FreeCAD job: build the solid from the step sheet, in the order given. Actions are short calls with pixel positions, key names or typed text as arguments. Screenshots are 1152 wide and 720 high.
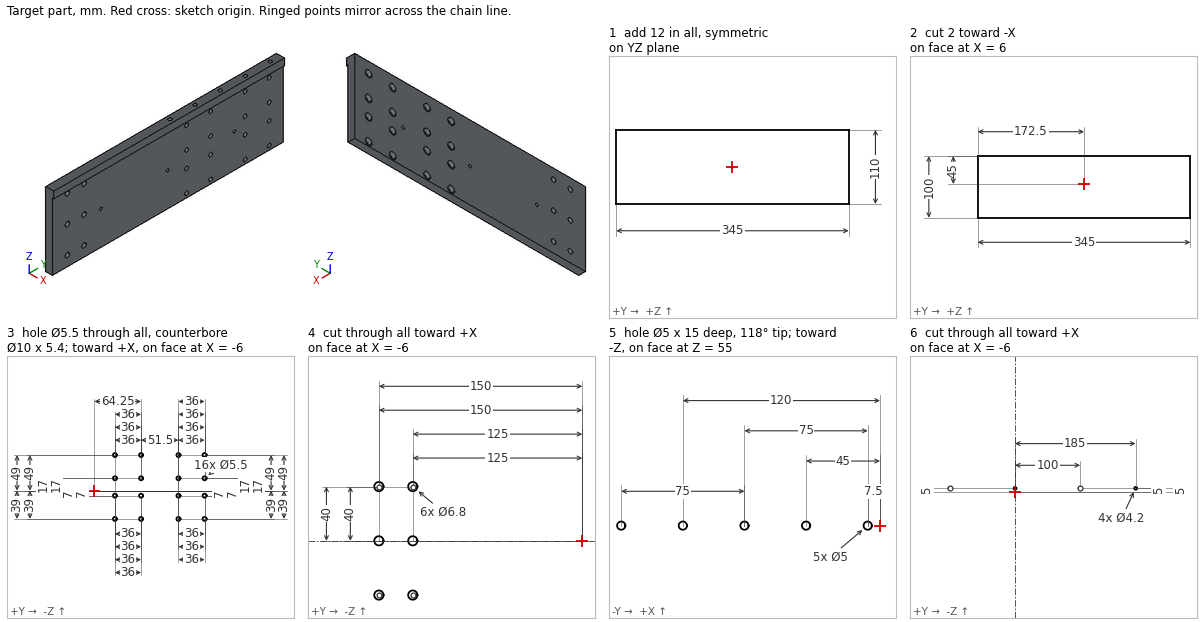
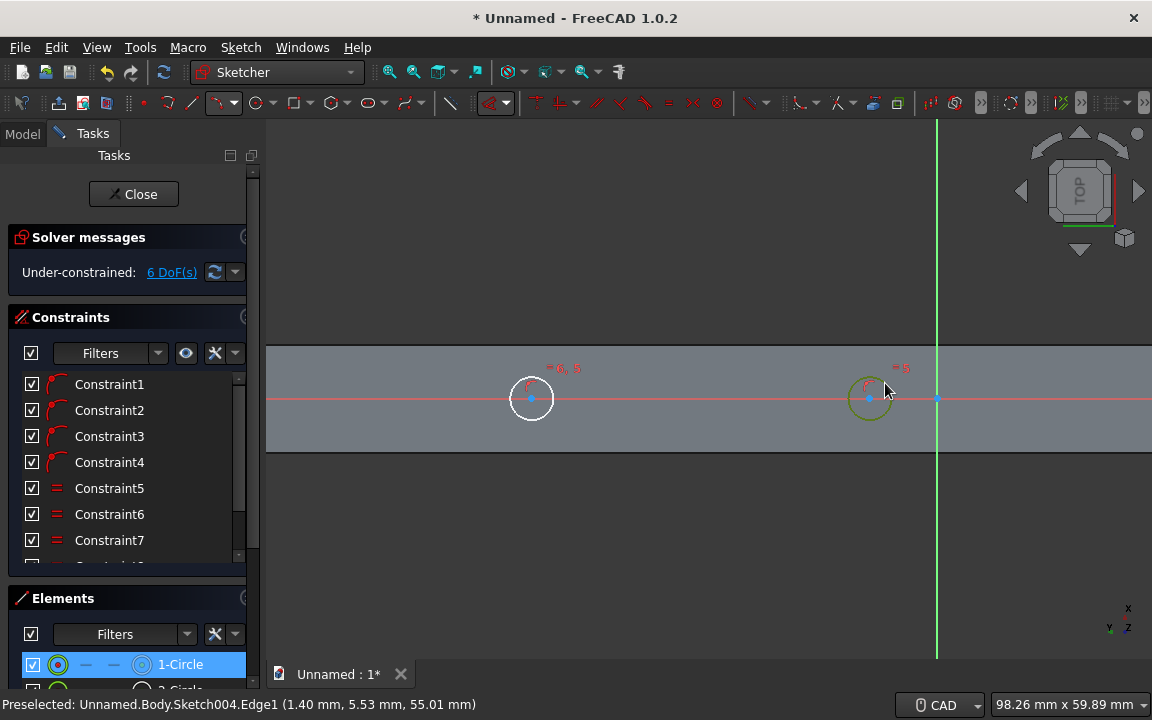
click(508, 104)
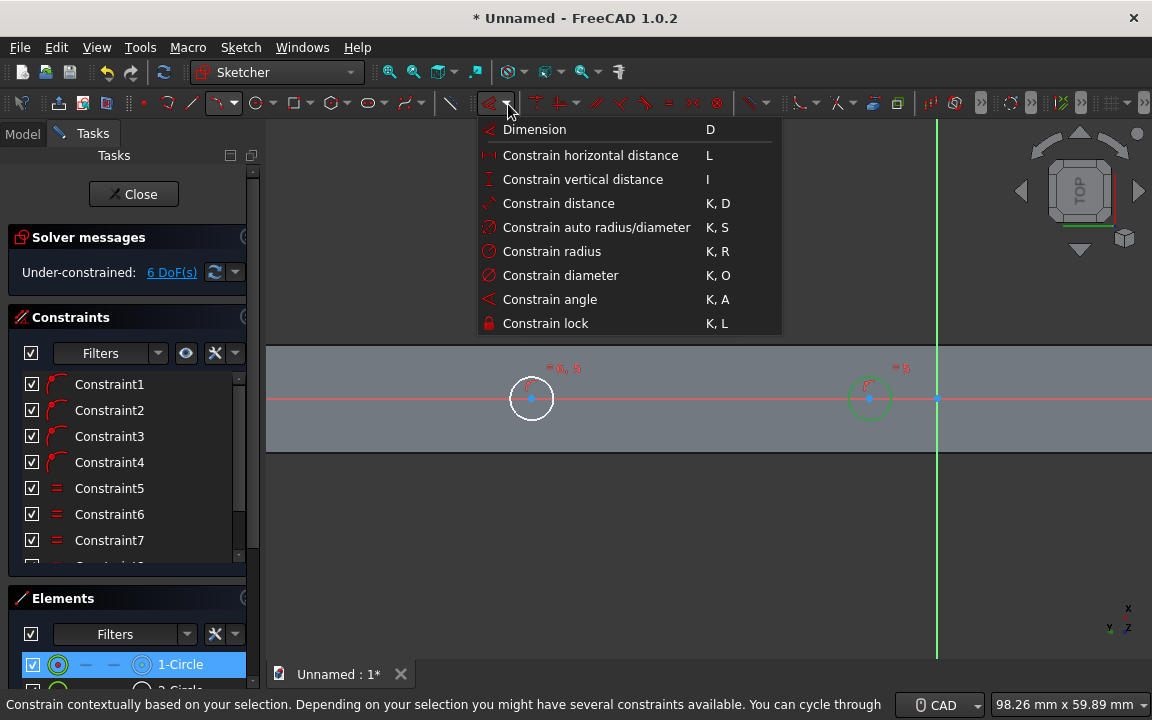
click(630, 275)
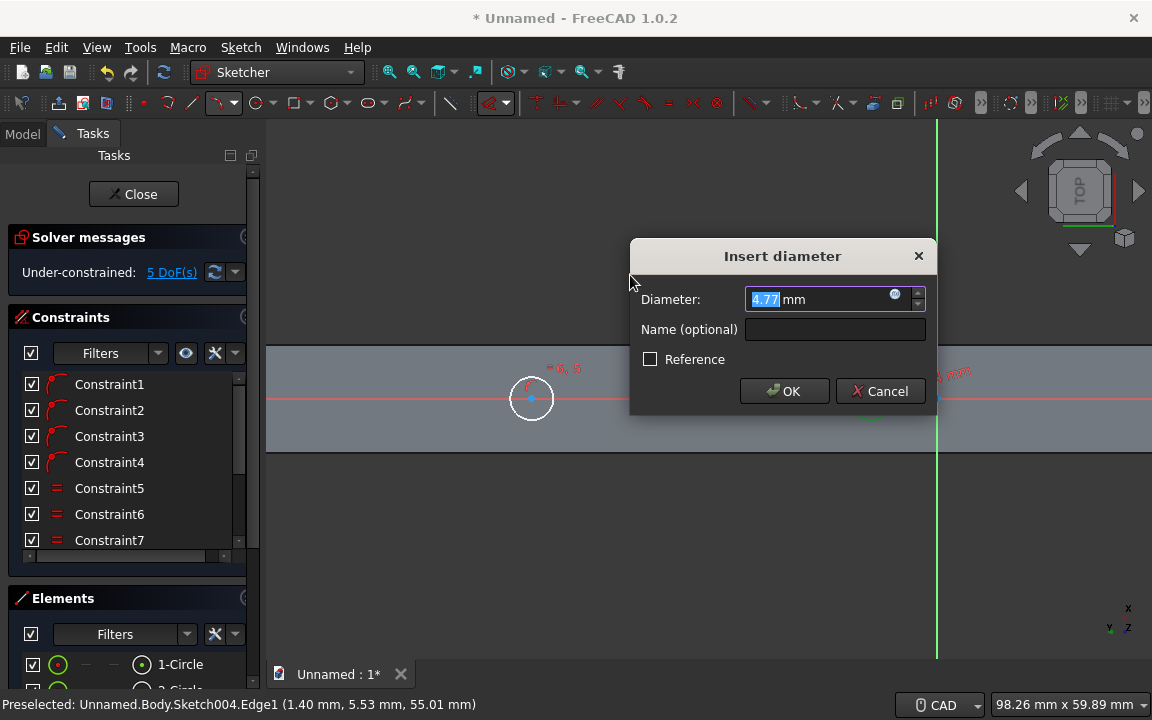
text(5)
key(Return)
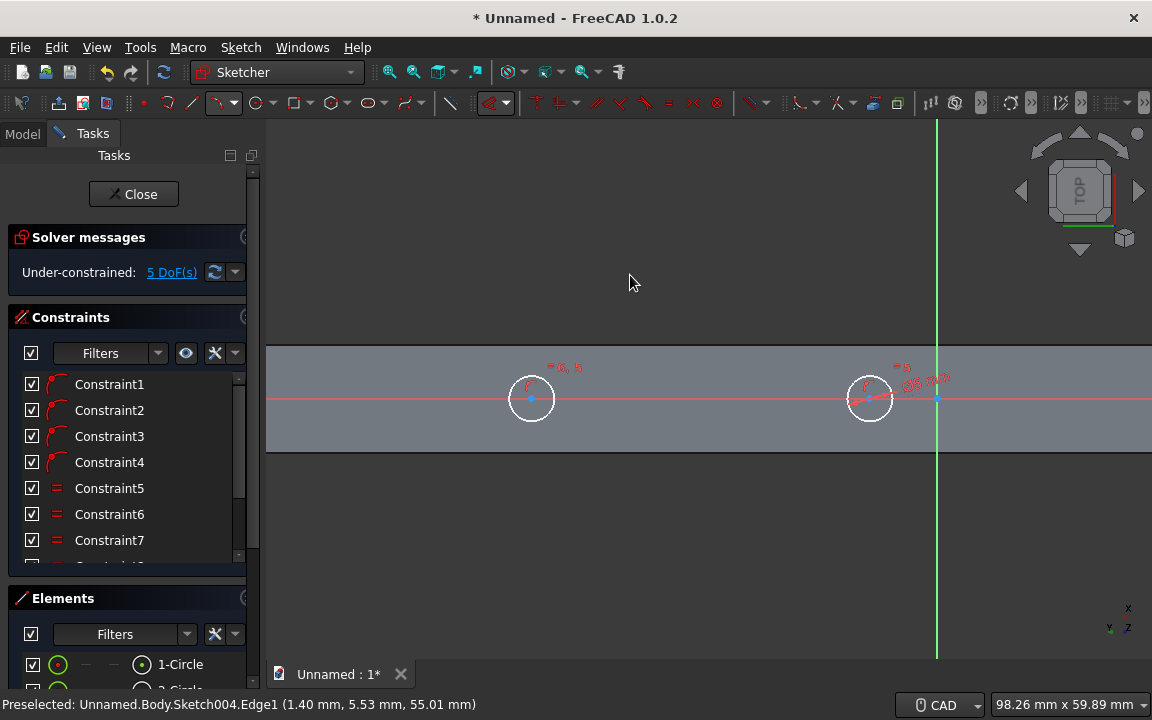
click(532, 399)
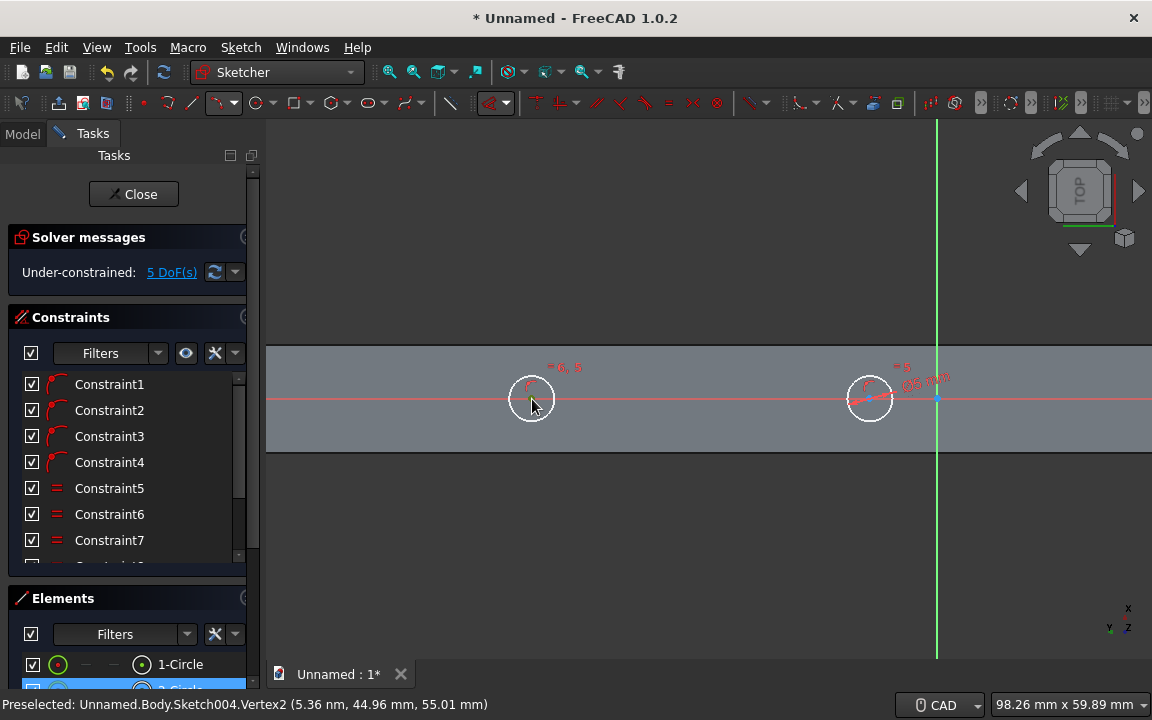
key(l)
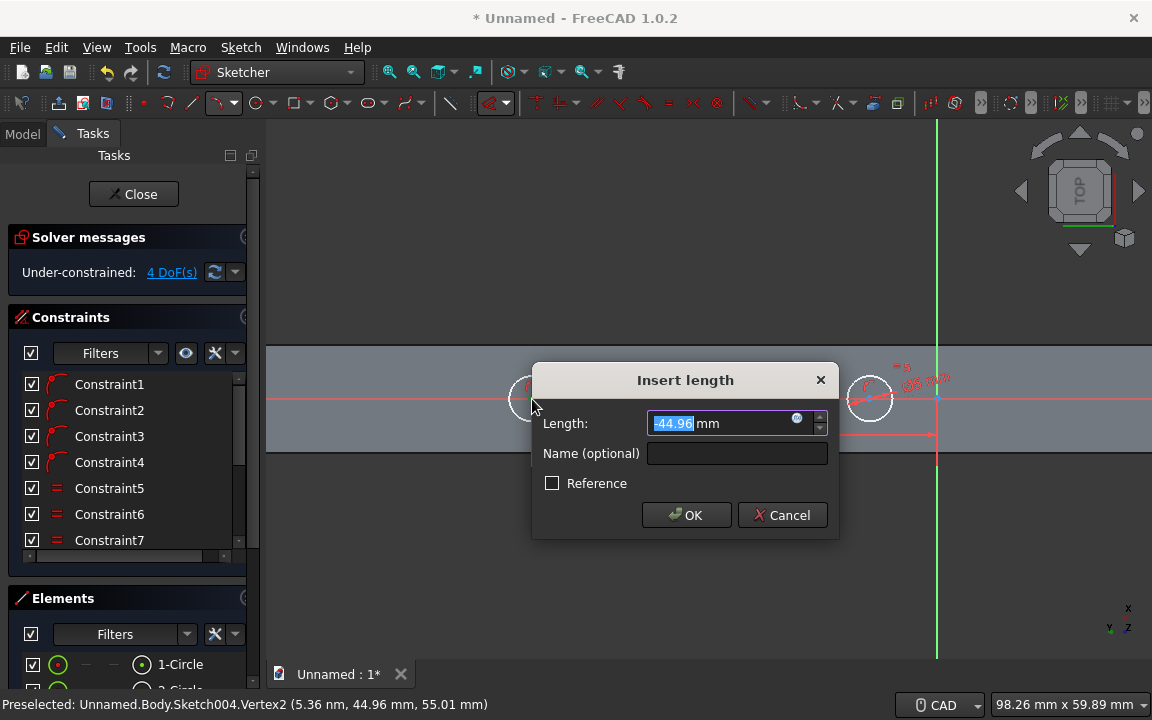
text(-45)
key(Return)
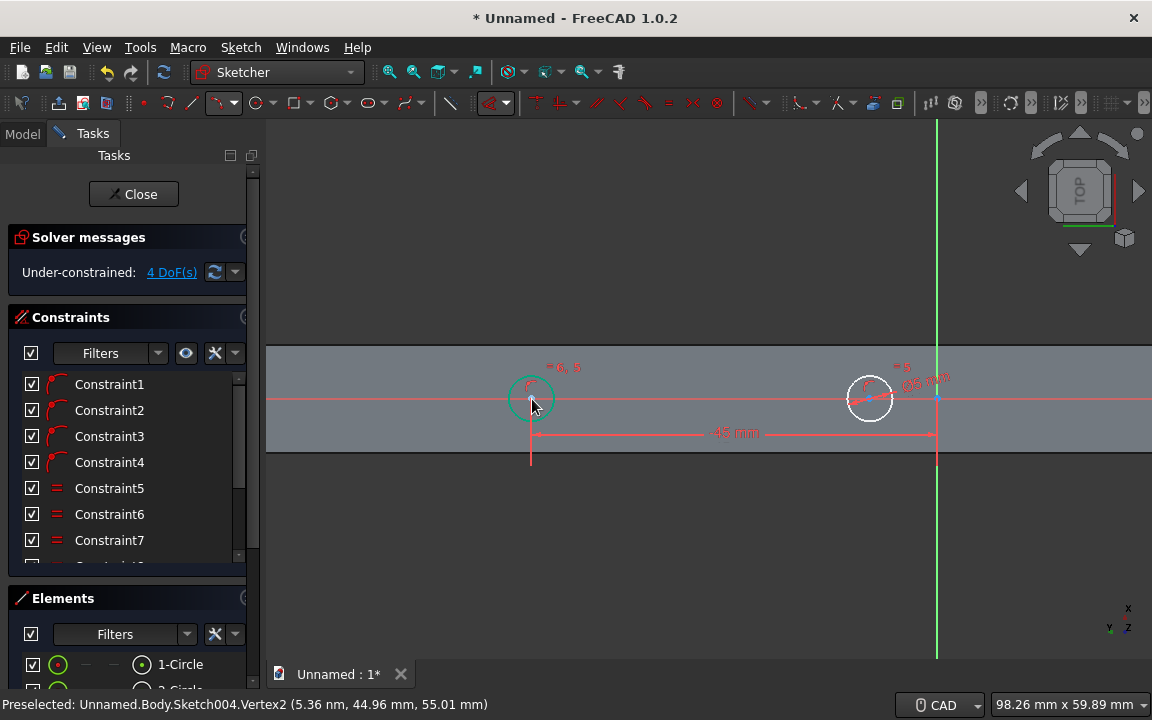
click(870, 399)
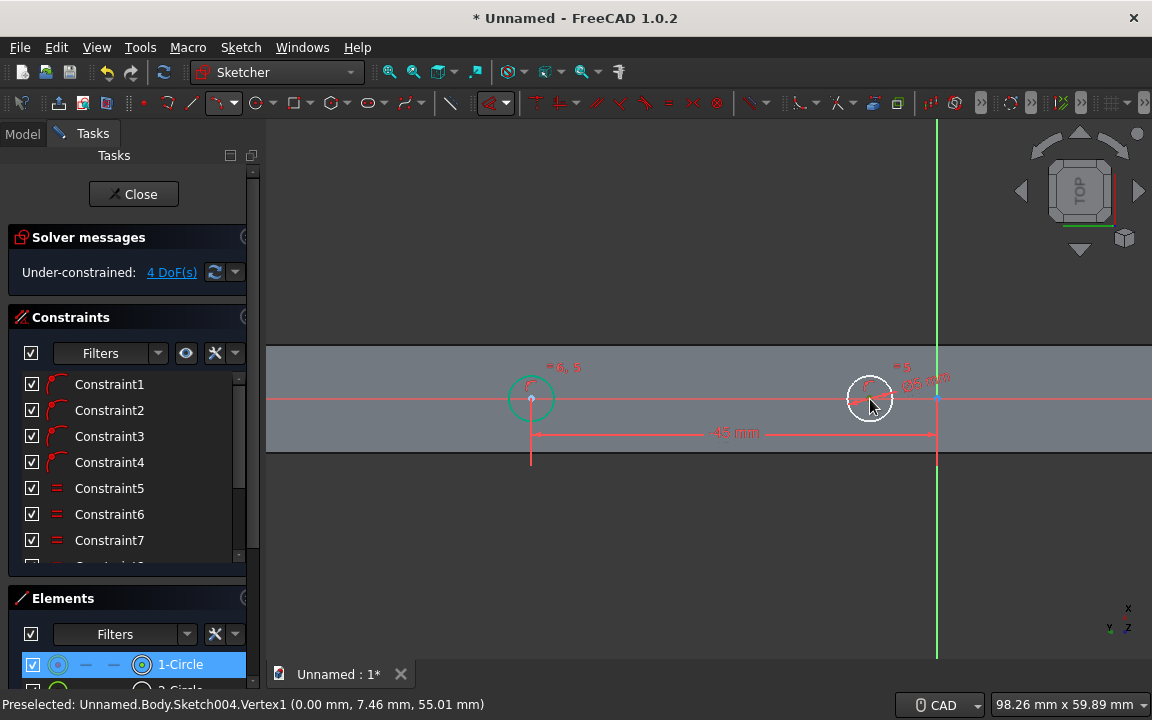
key(l)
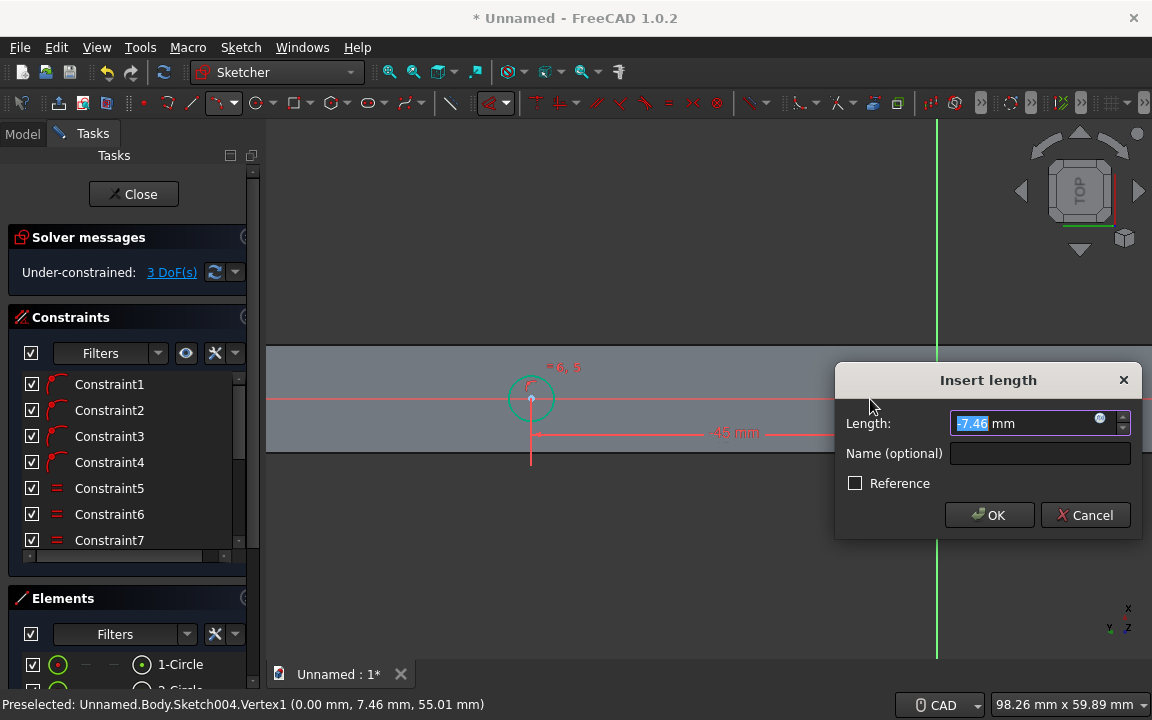
text(-7.5)
key(Return)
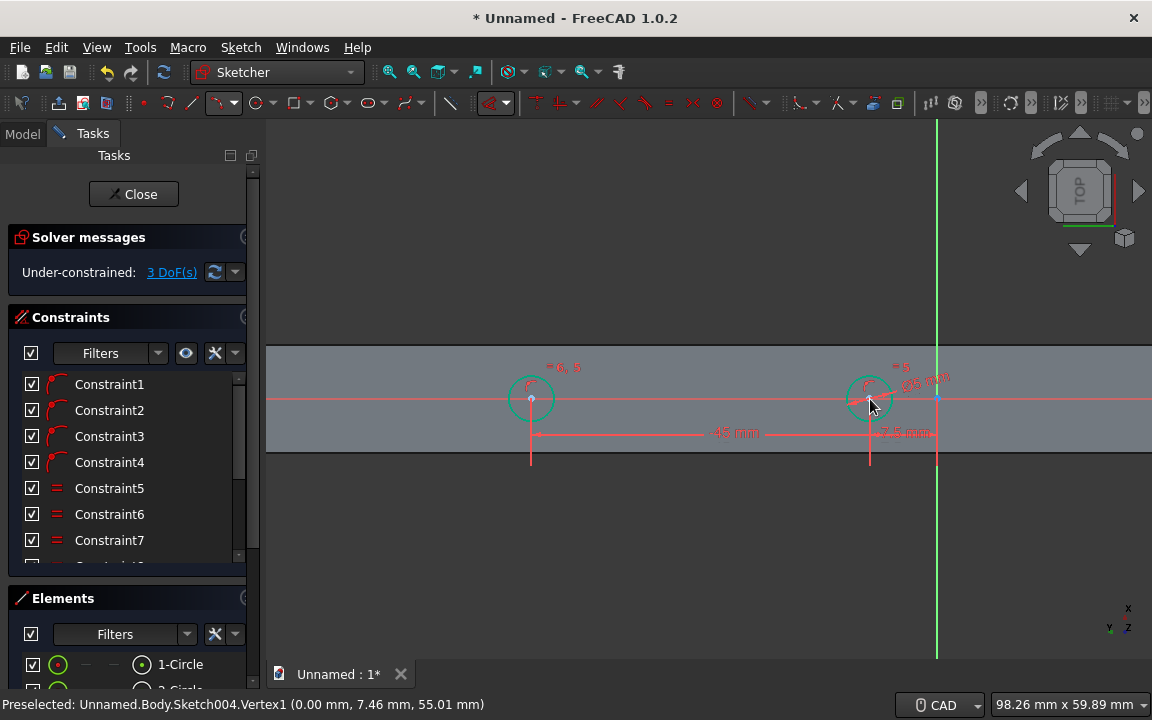
scroll(888, 383, down, 5)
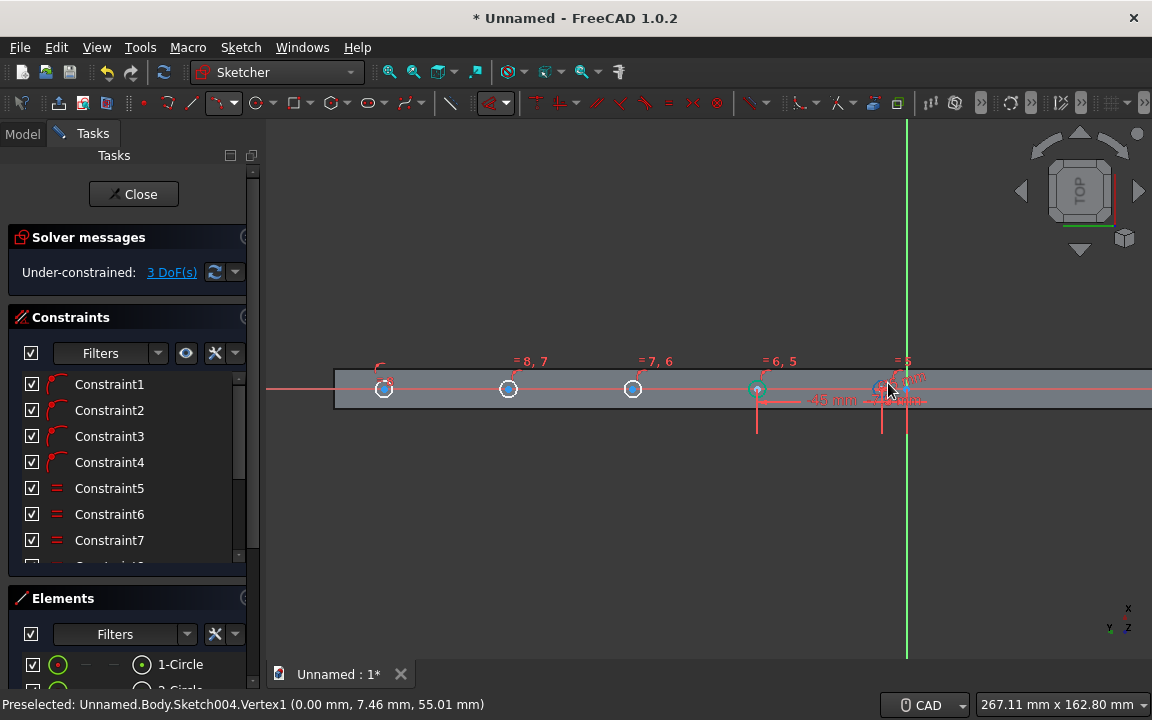
click(509, 389)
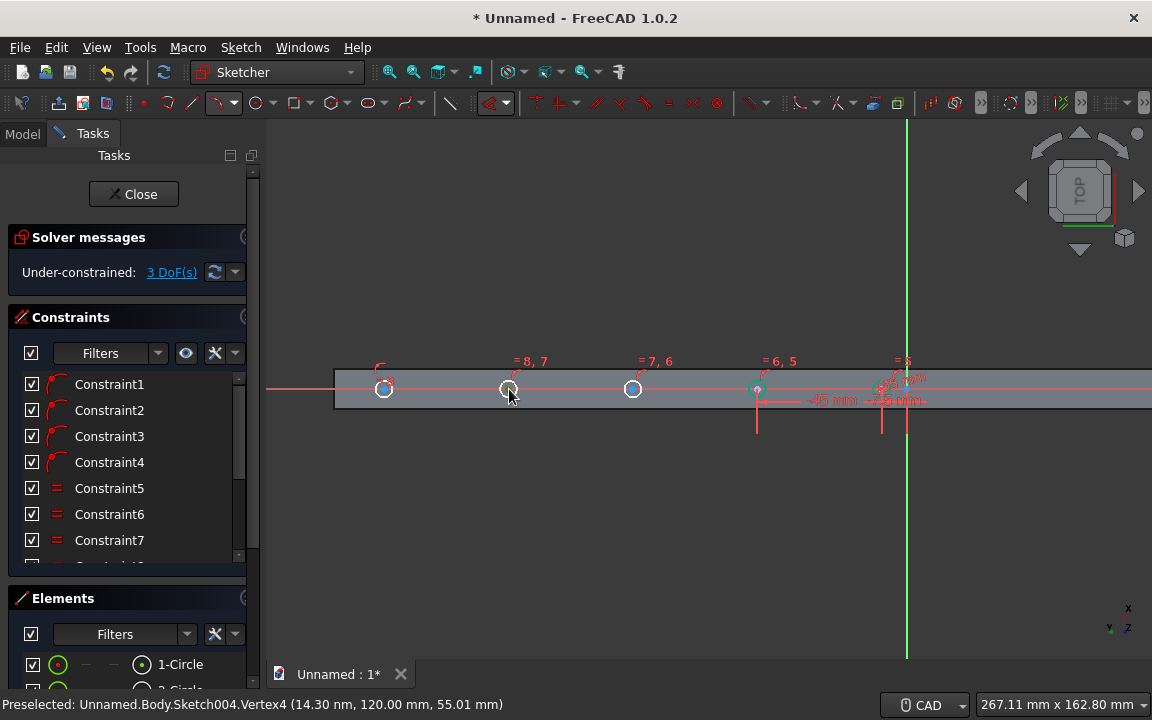
key(l)